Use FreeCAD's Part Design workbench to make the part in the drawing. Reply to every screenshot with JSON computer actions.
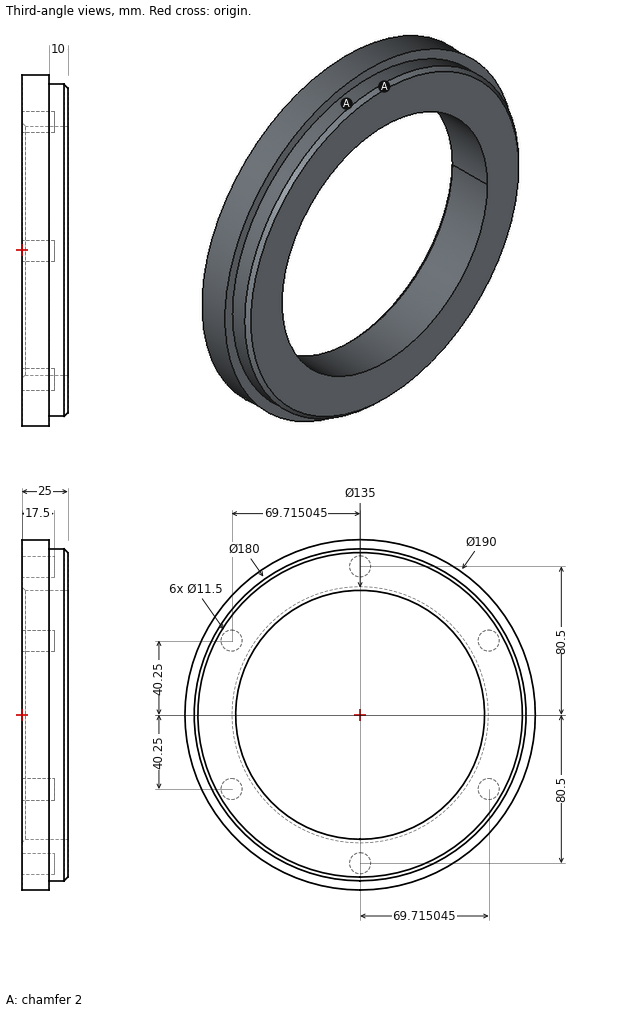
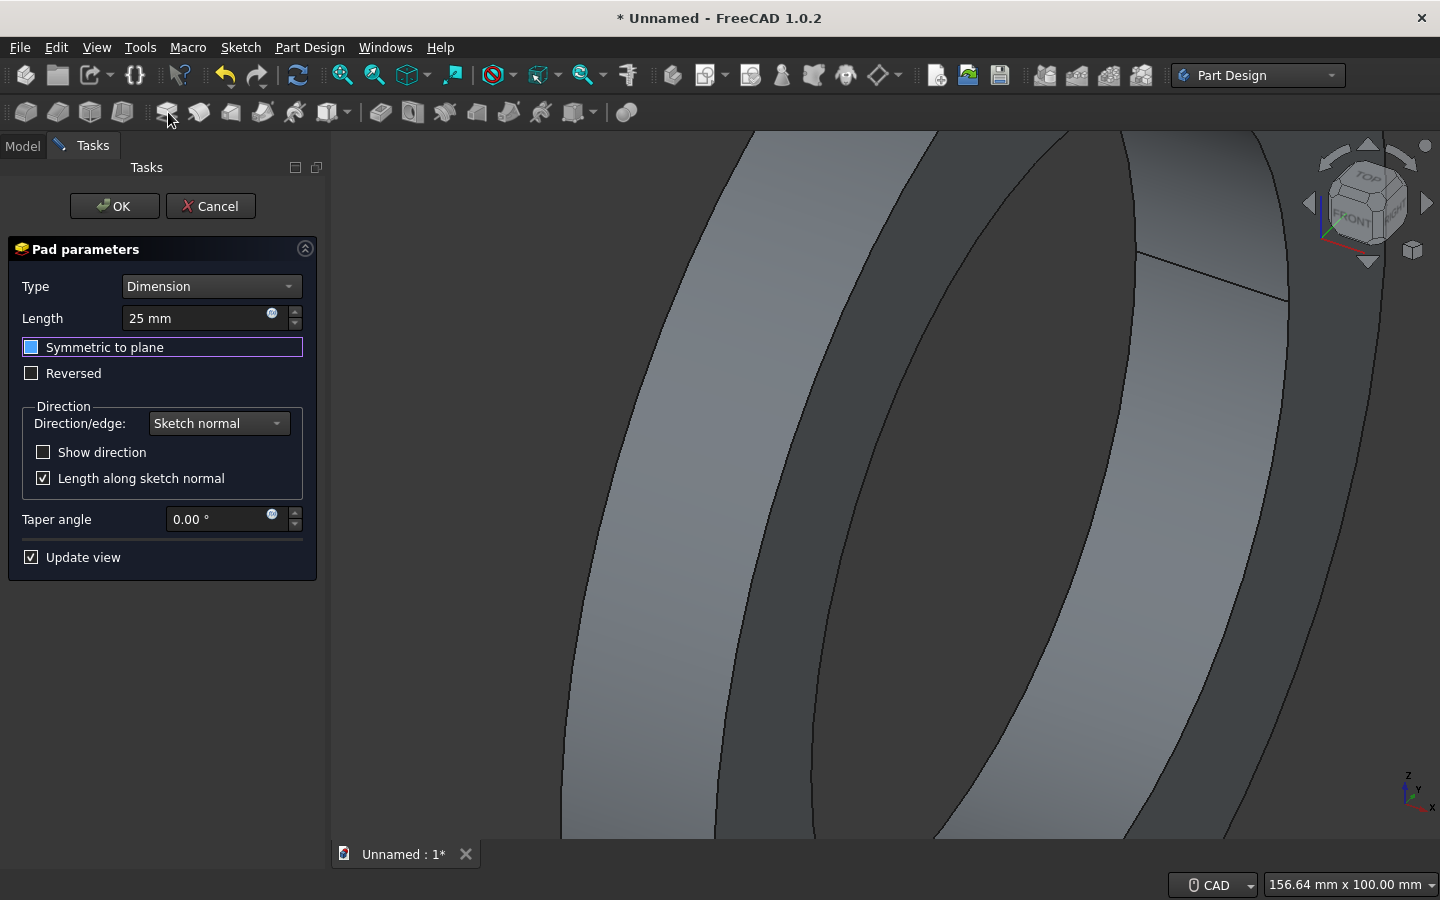
{"action": "left_click", "coordinate": [115, 206]}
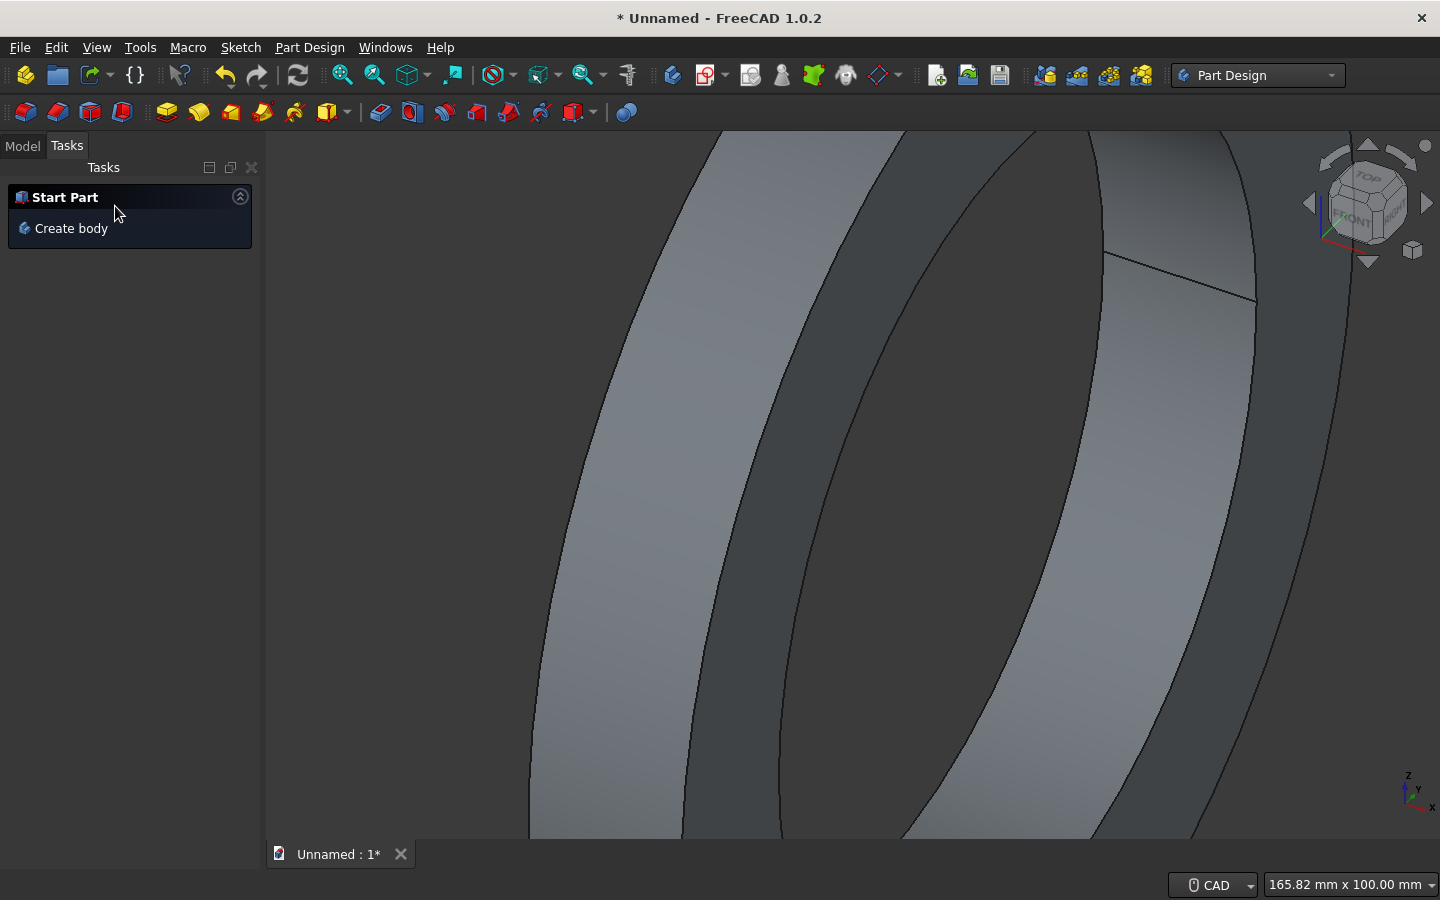
{"action": "left_click", "coordinate": [344, 76]}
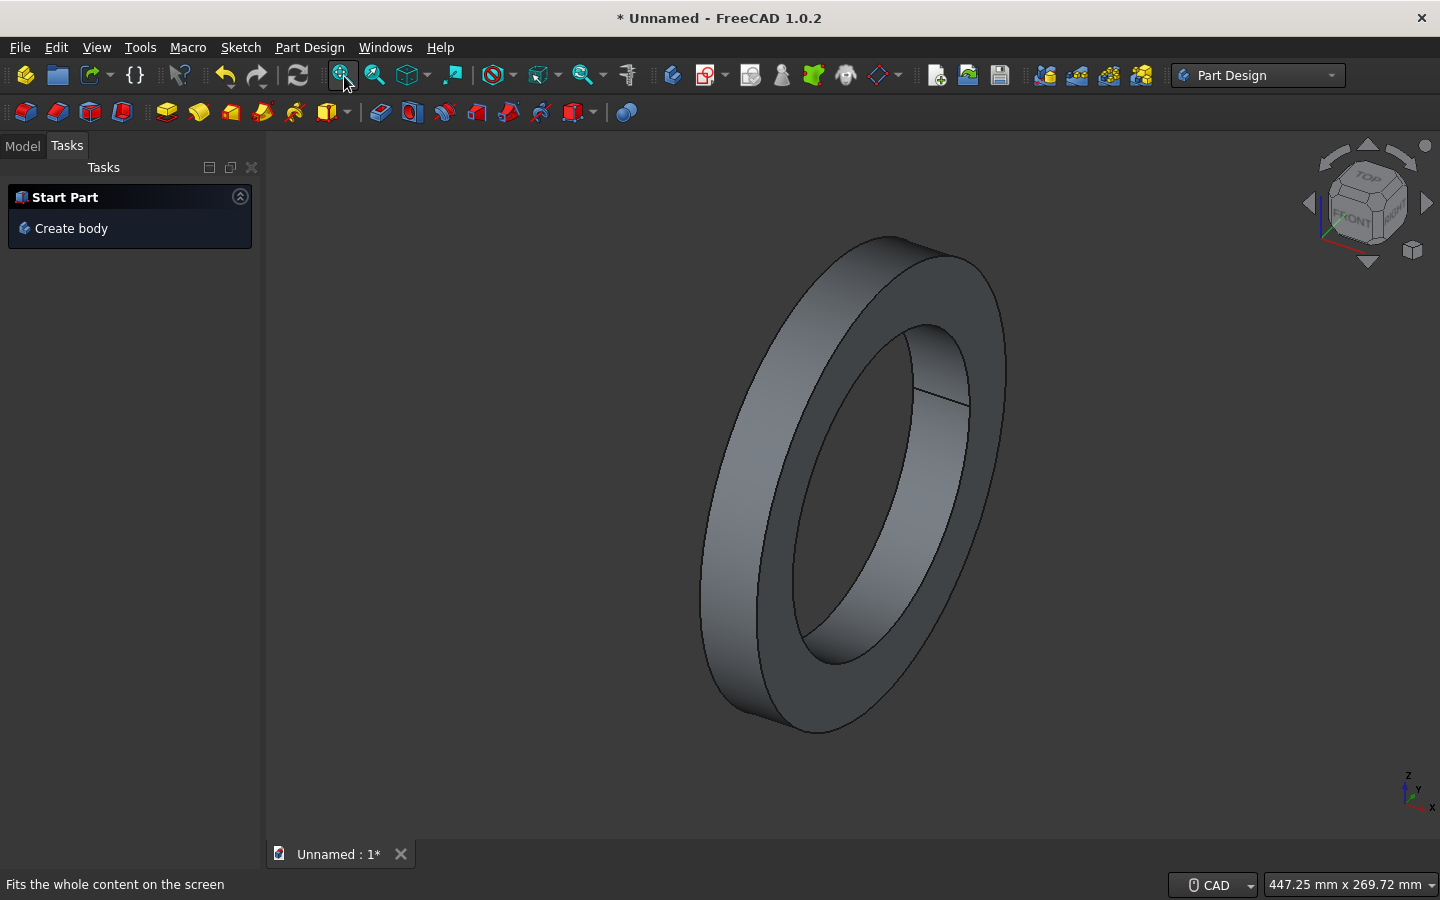
{"action": "left_click", "coordinate": [23, 145]}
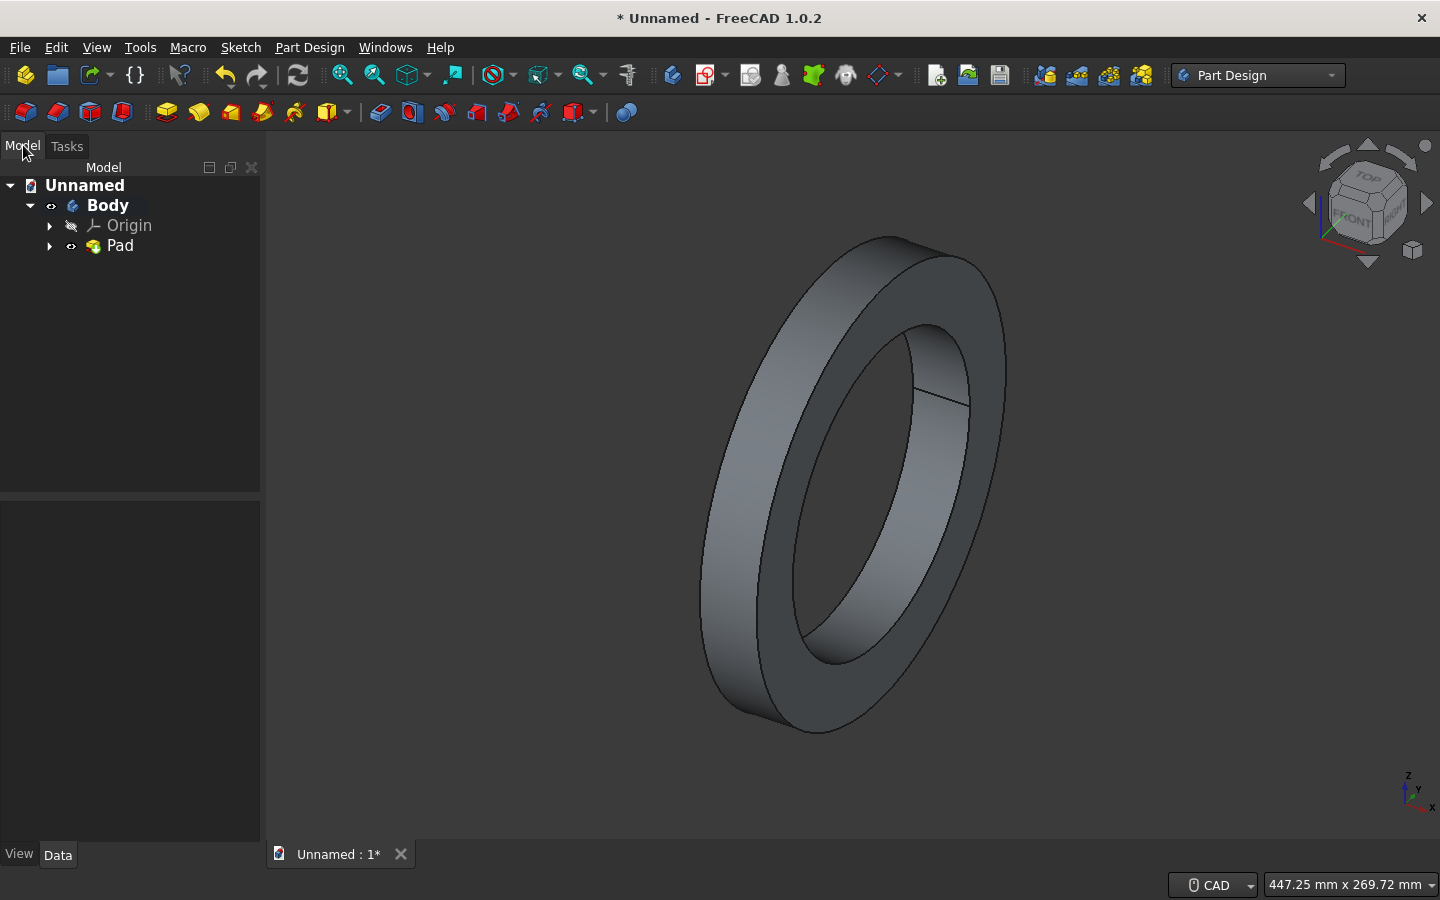
{"action": "left_click", "coordinate": [50, 226]}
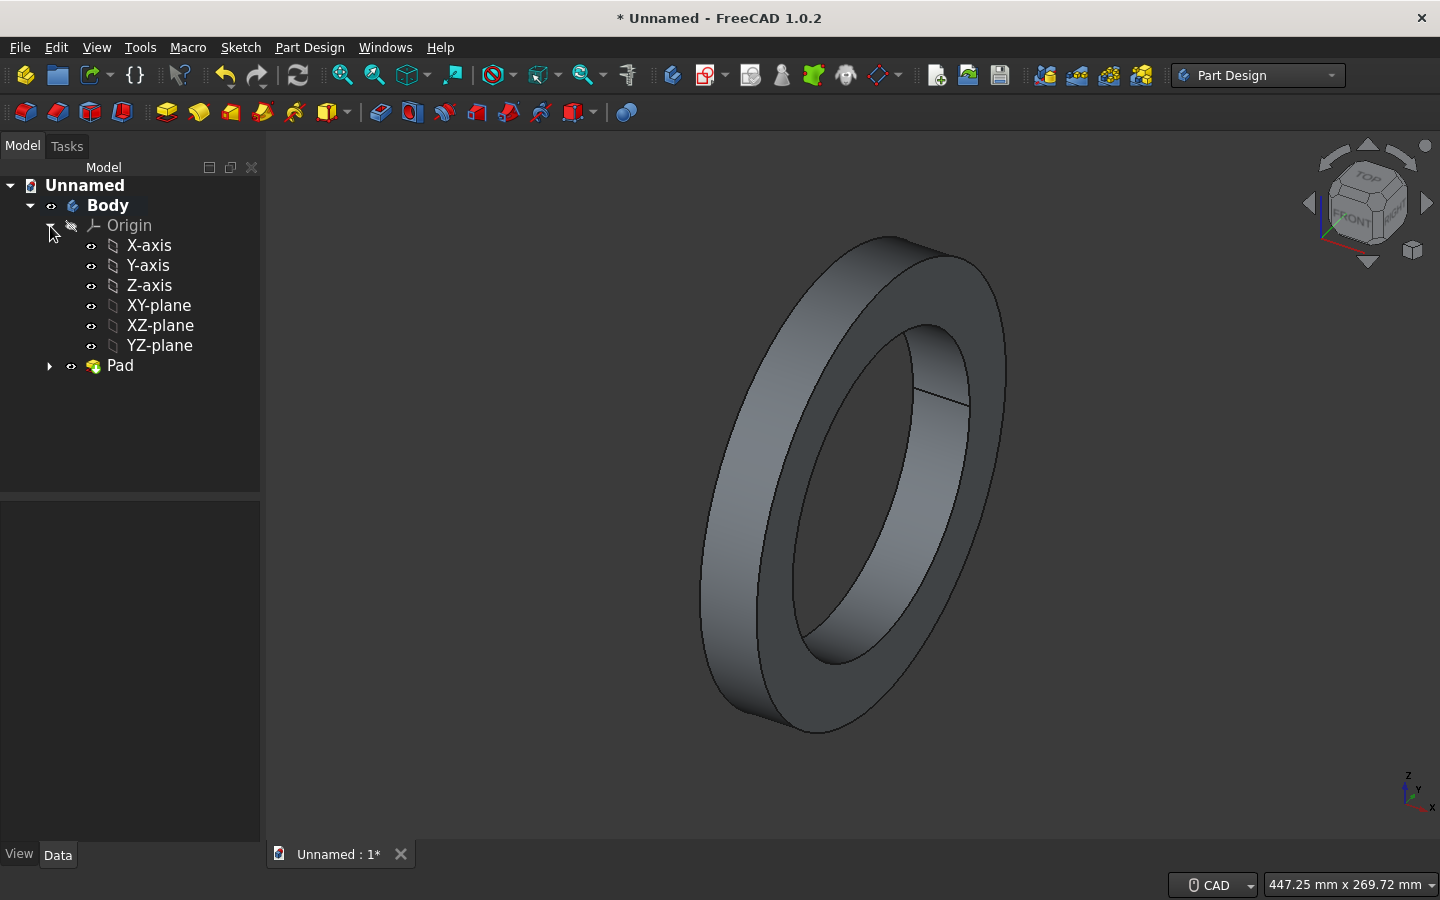
{"action": "left_click", "coordinate": [136, 346]}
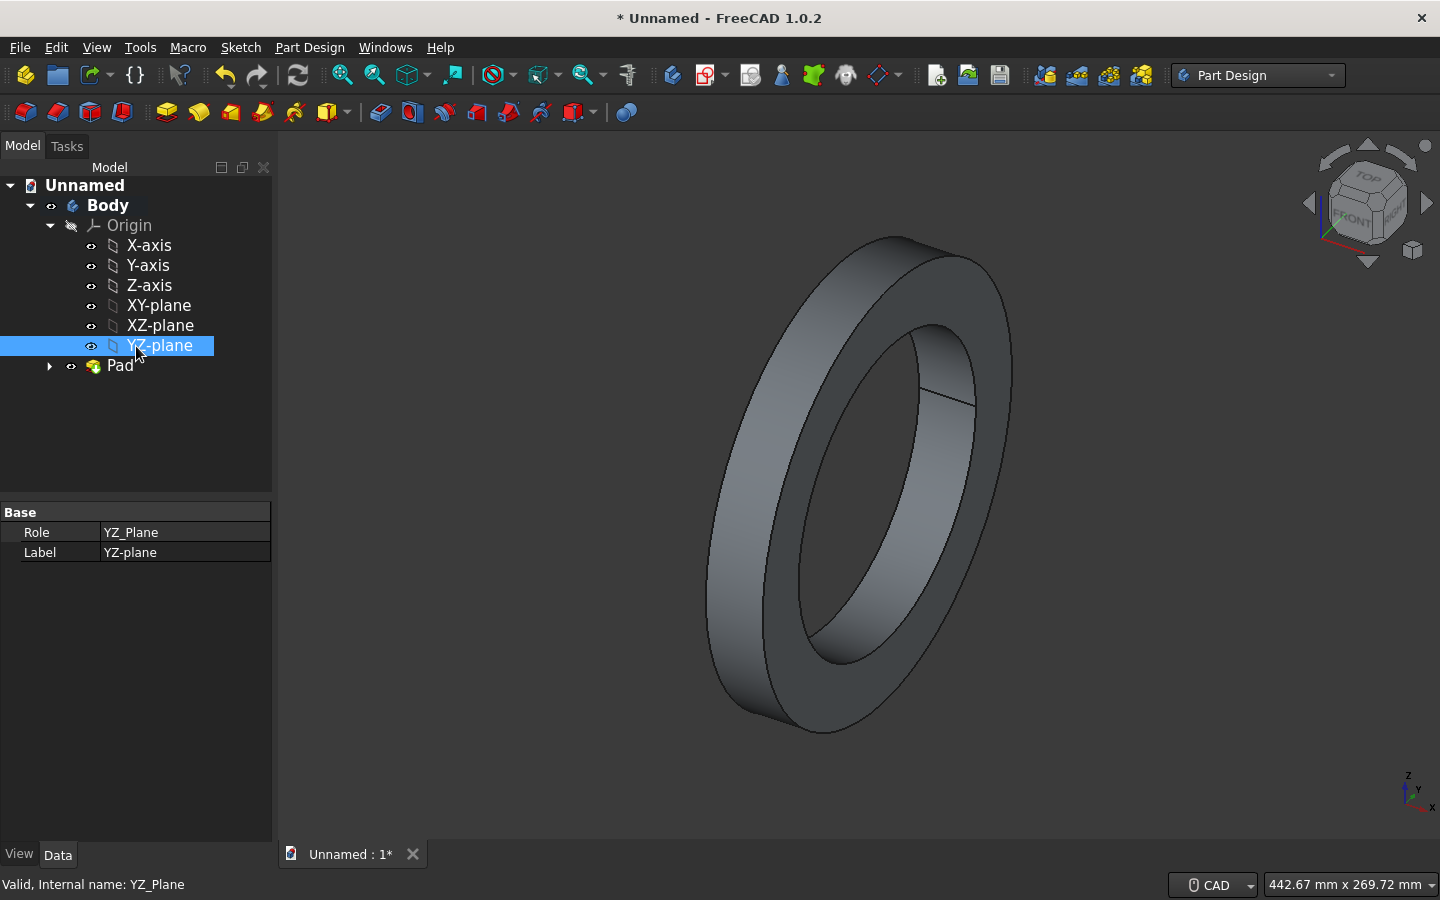
{"action": "left_click", "coordinate": [878, 76]}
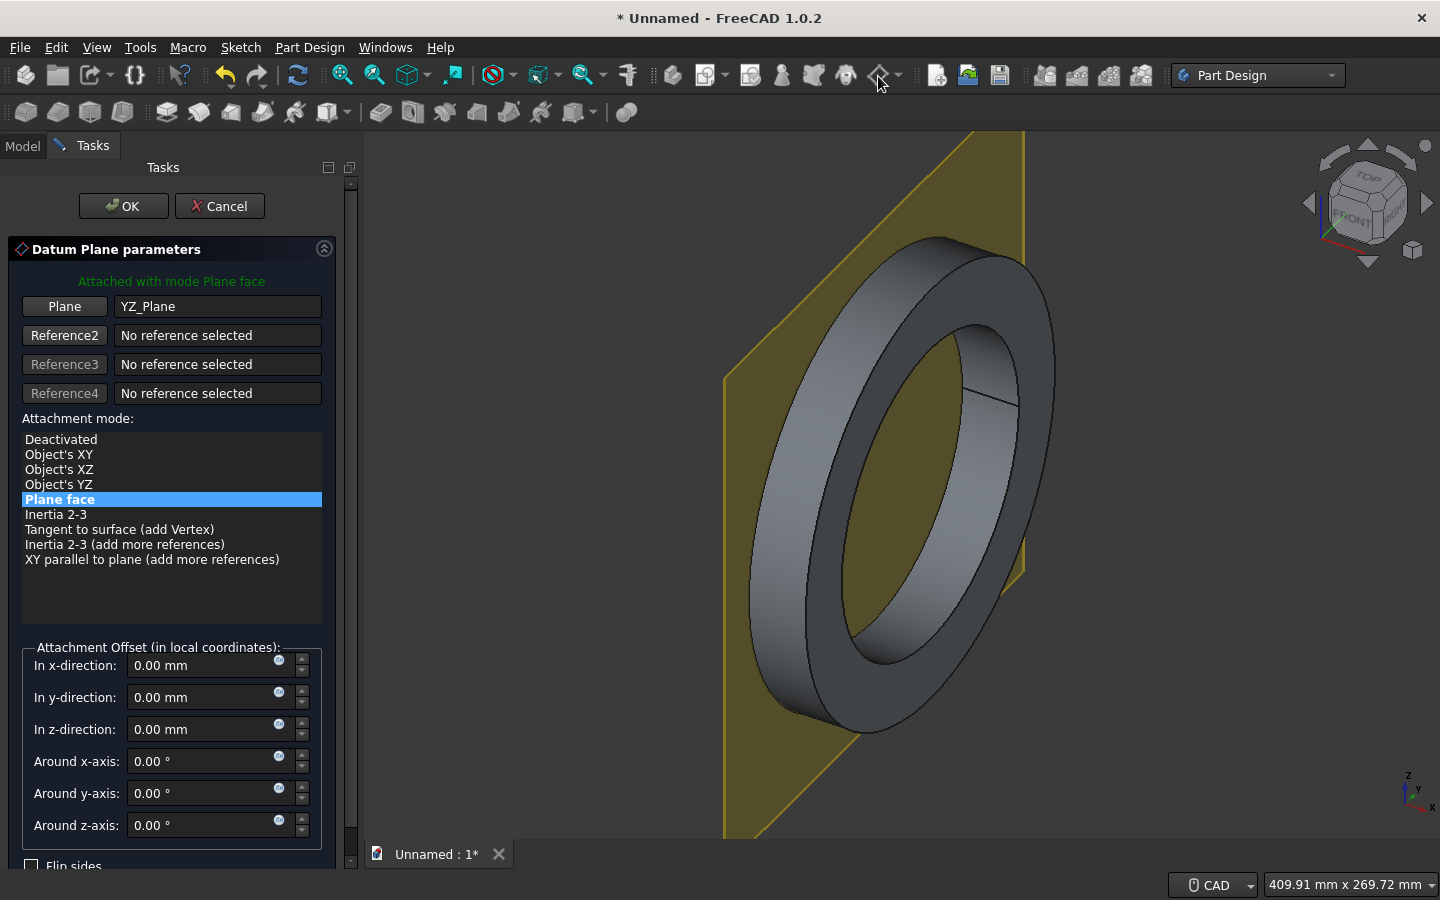
{"action": "triple_click", "coordinate": [210, 729]}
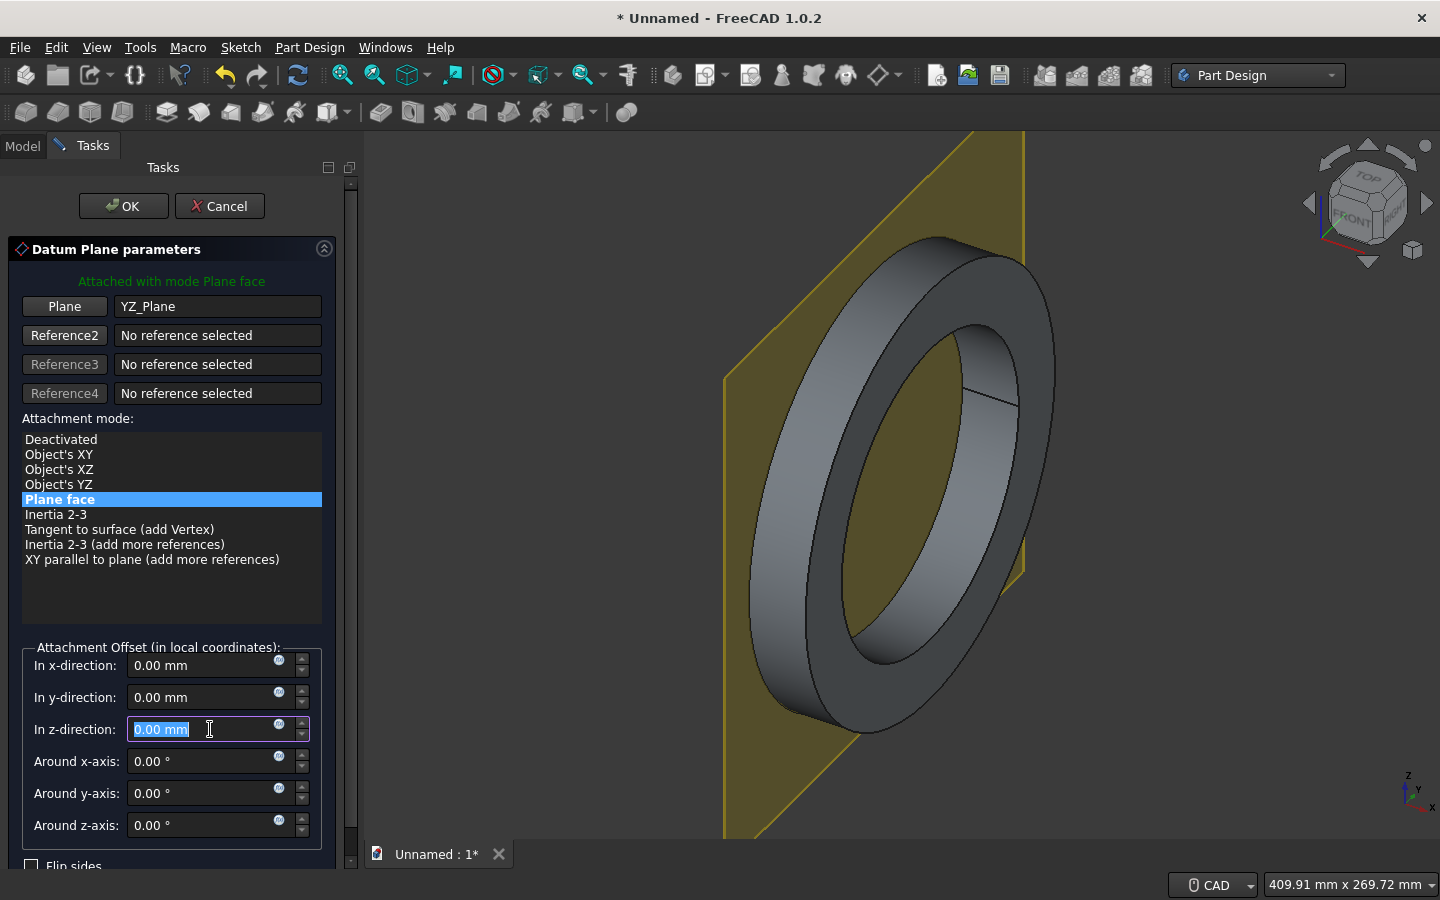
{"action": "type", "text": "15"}
{"action": "key", "text": "Tab"}